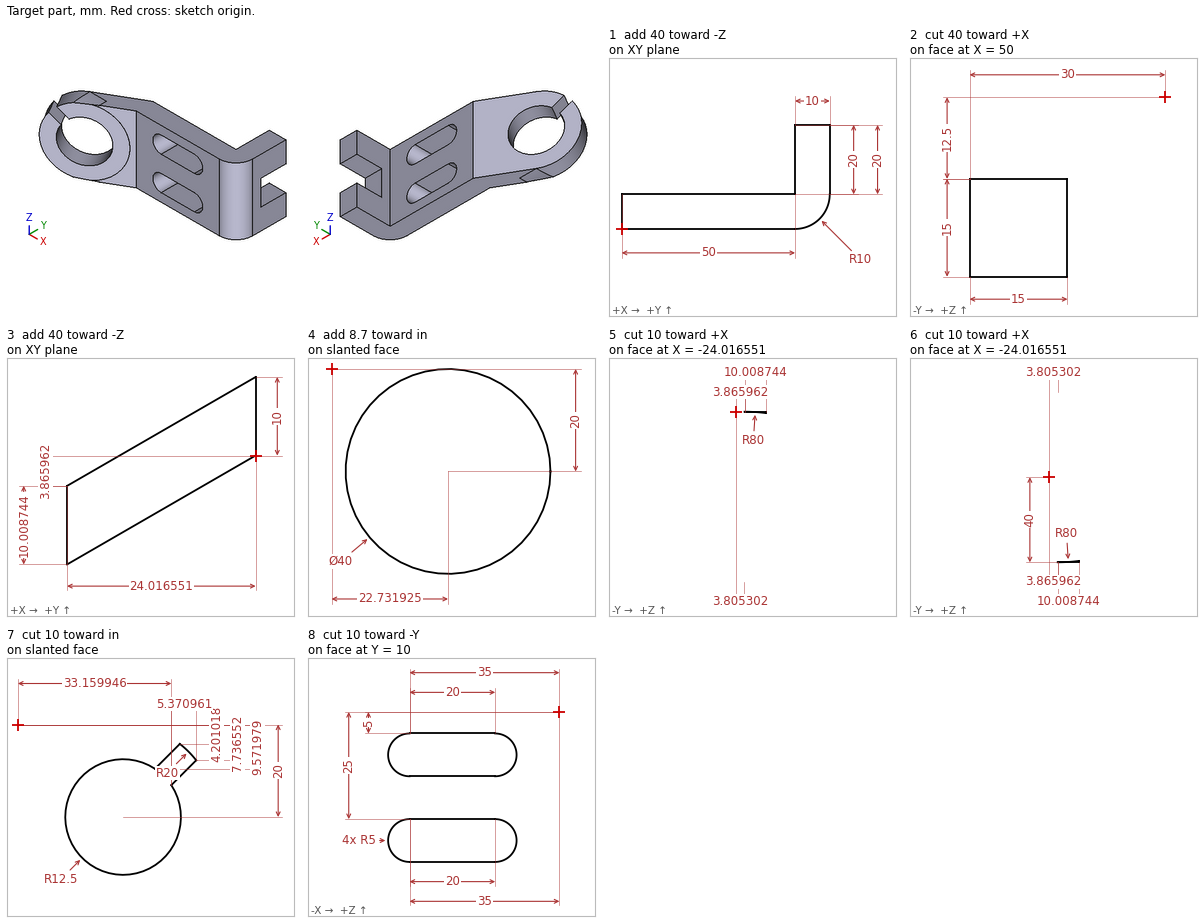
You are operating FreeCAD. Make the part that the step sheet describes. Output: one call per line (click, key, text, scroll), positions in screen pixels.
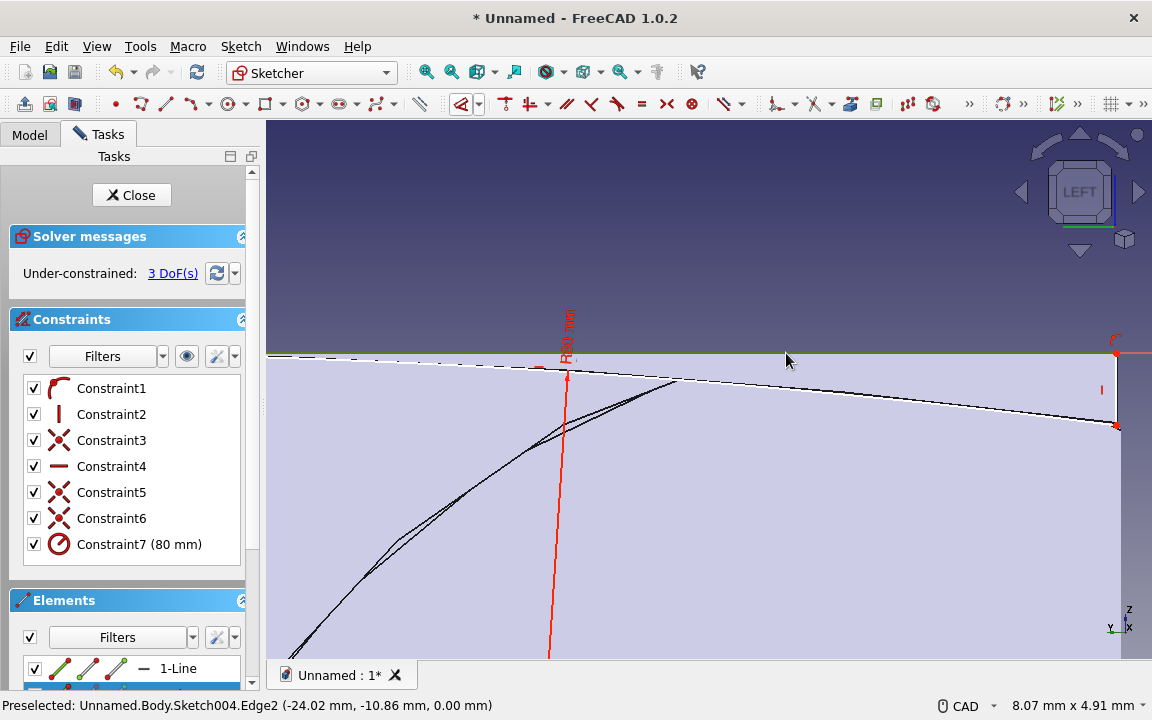
key(l)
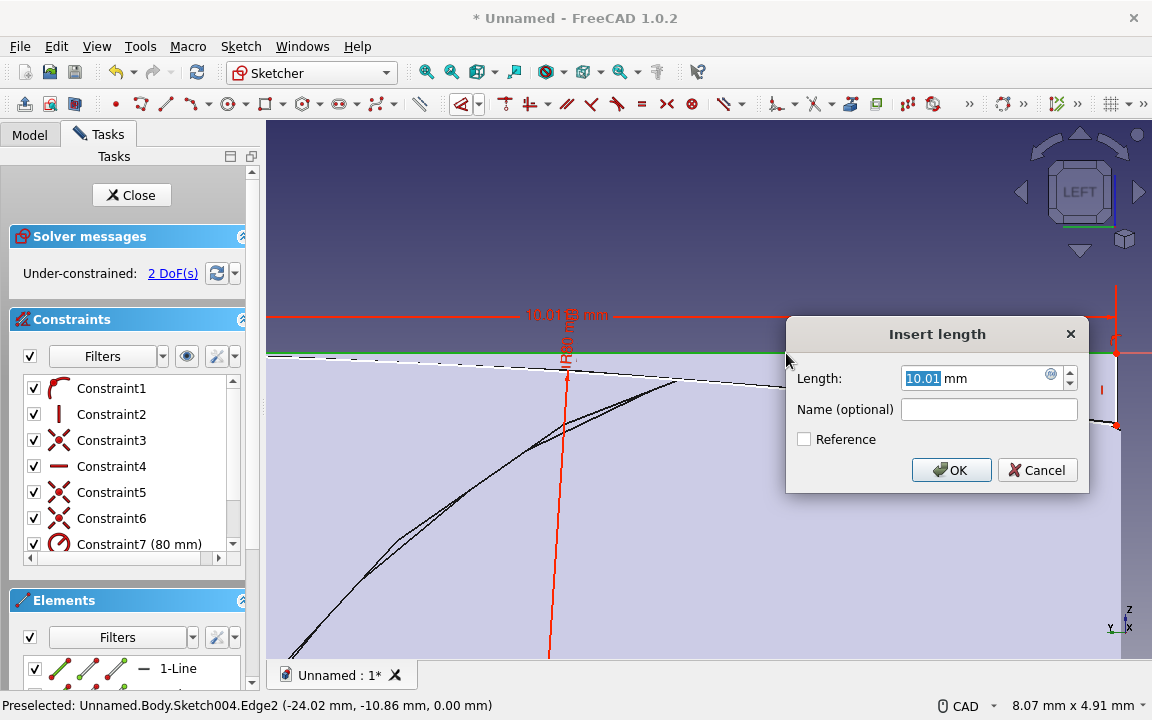
text(10.008744)
key(Return)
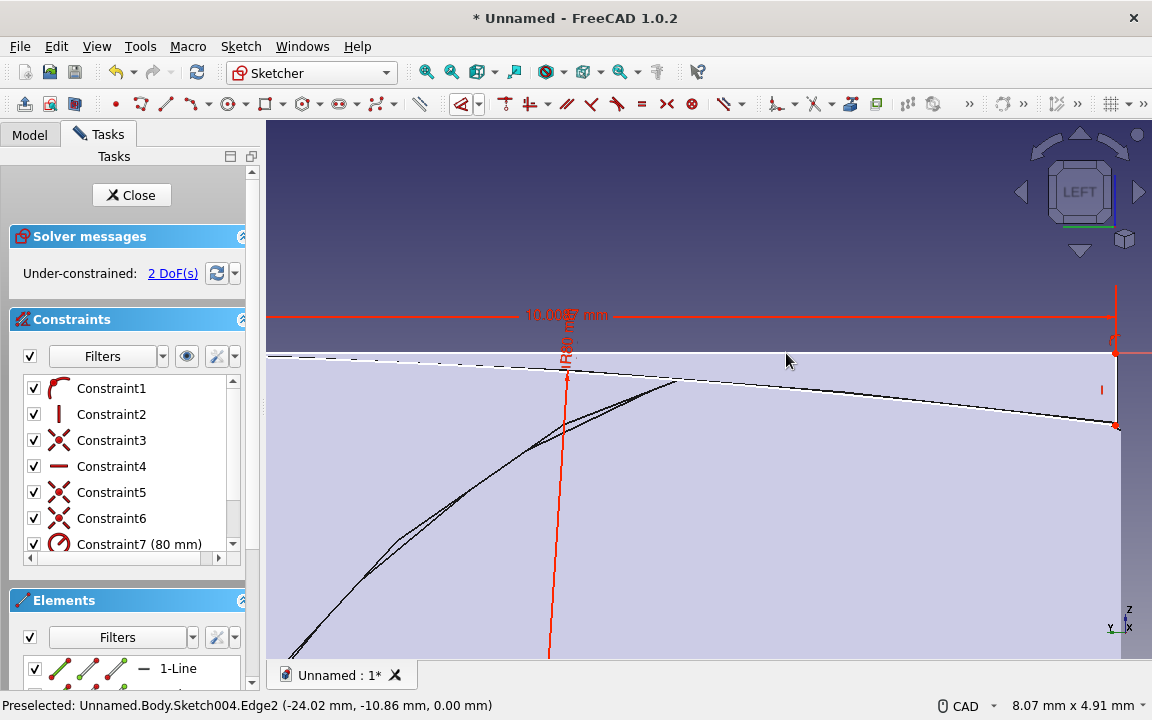
scroll(764, 390, down, 6)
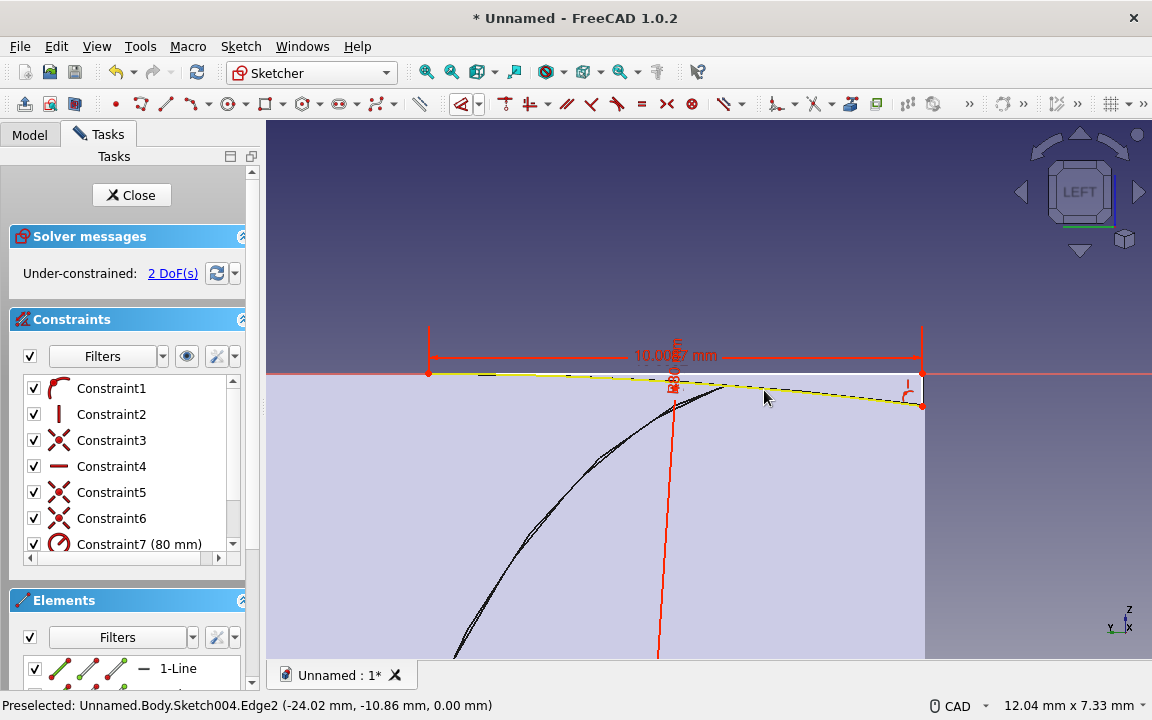
click(539, 379)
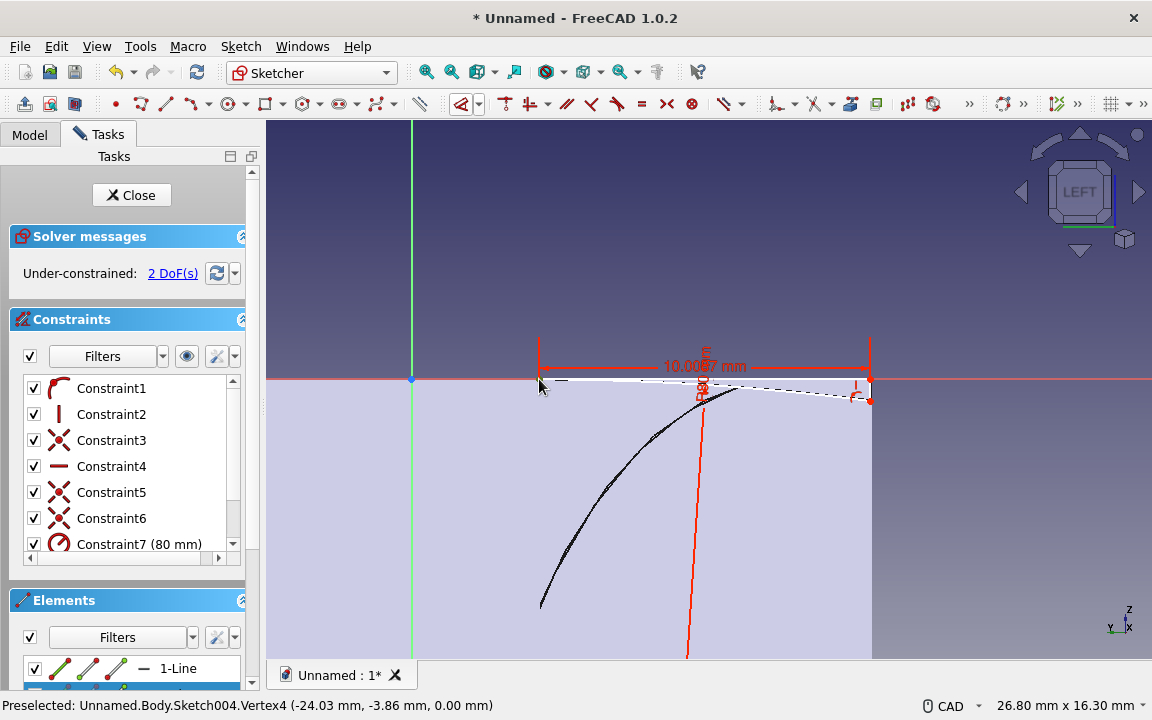
click(478, 104)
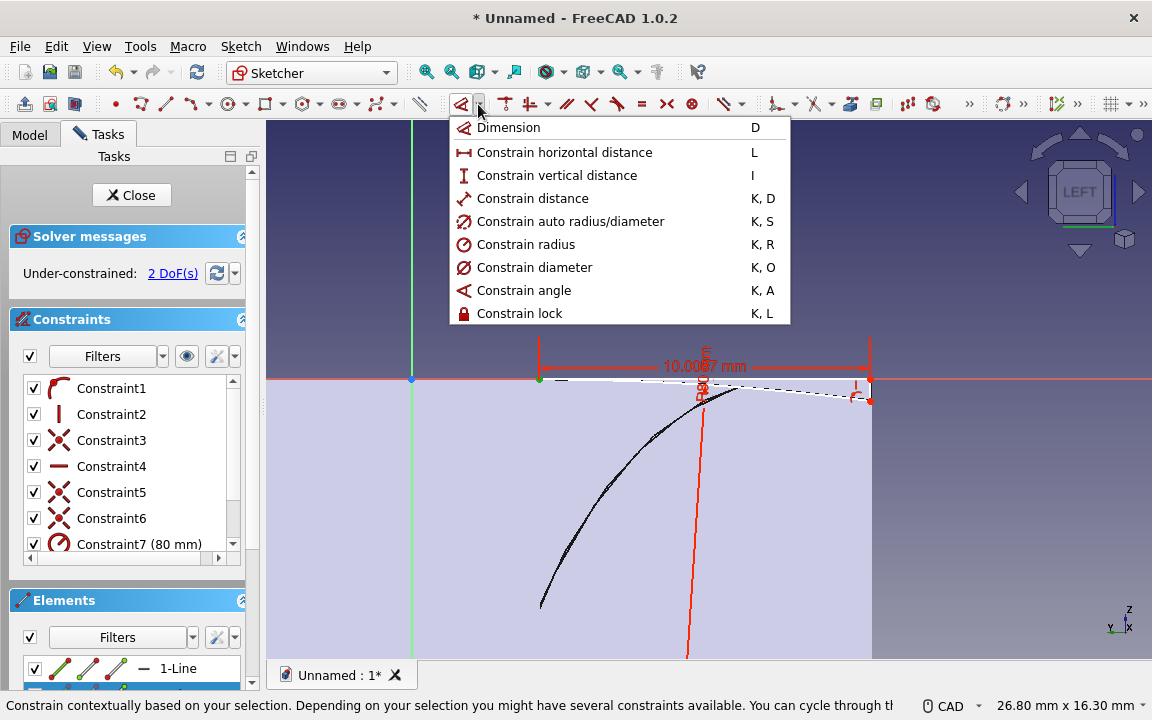
click(620, 152)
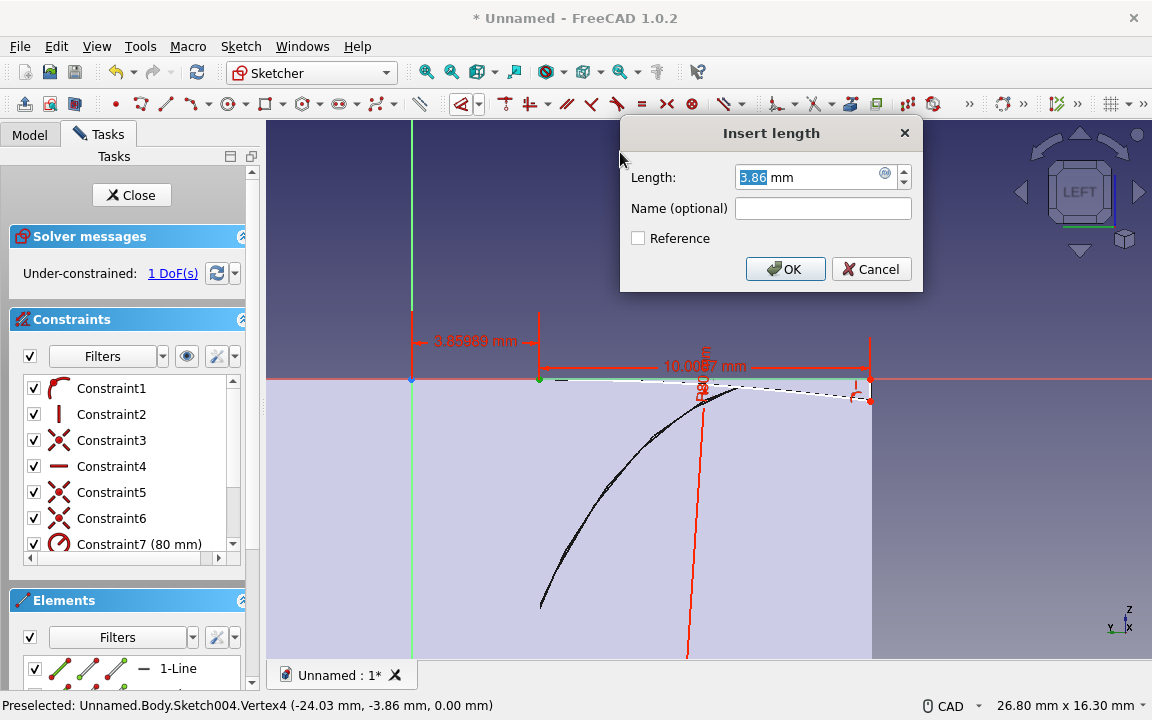
text(3.865962)
key(Return)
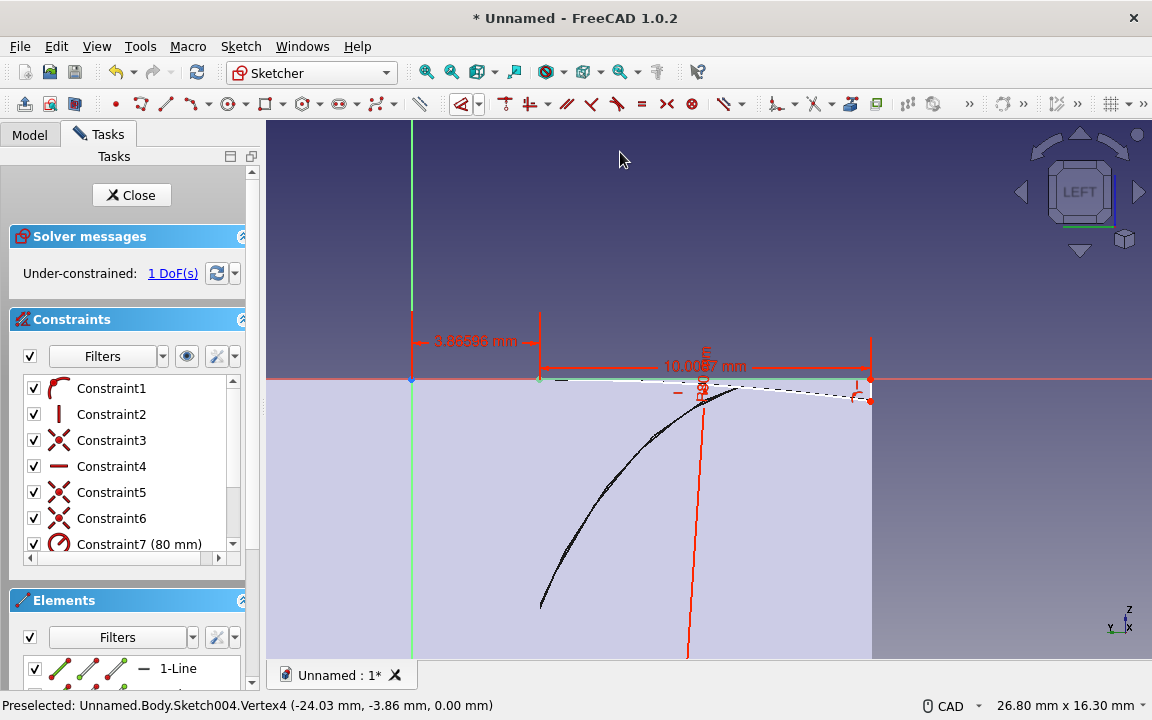
scroll(640, 184, down, 10)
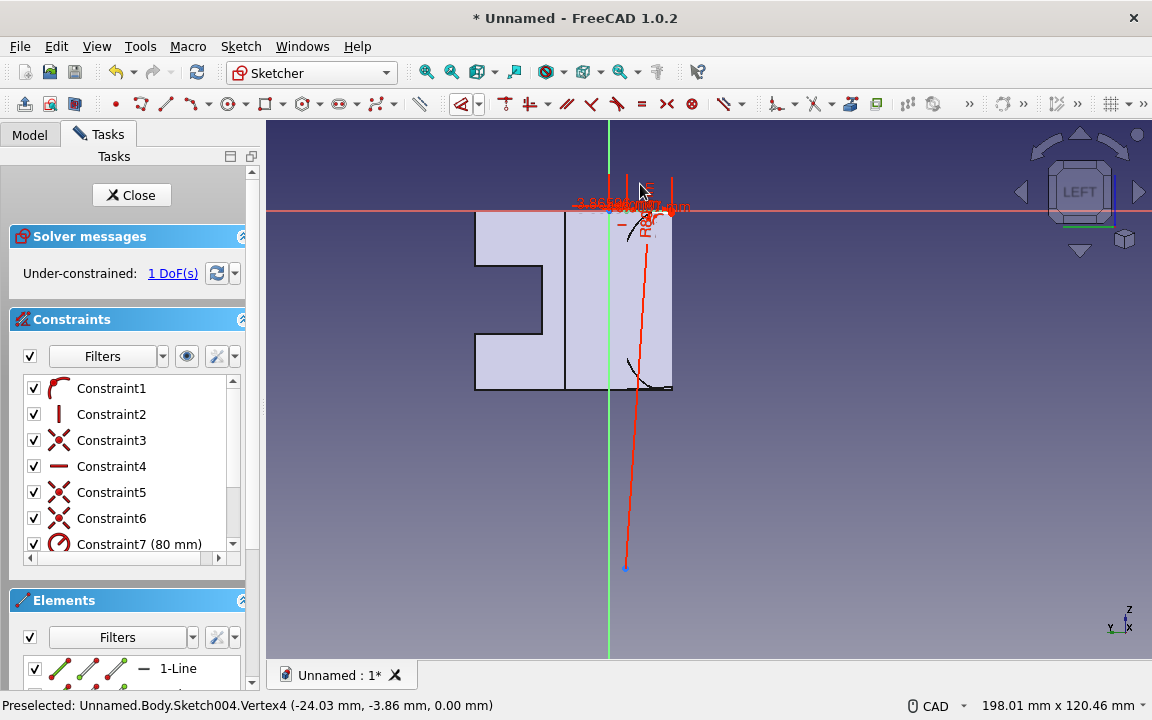
scroll(626, 568, up, 5)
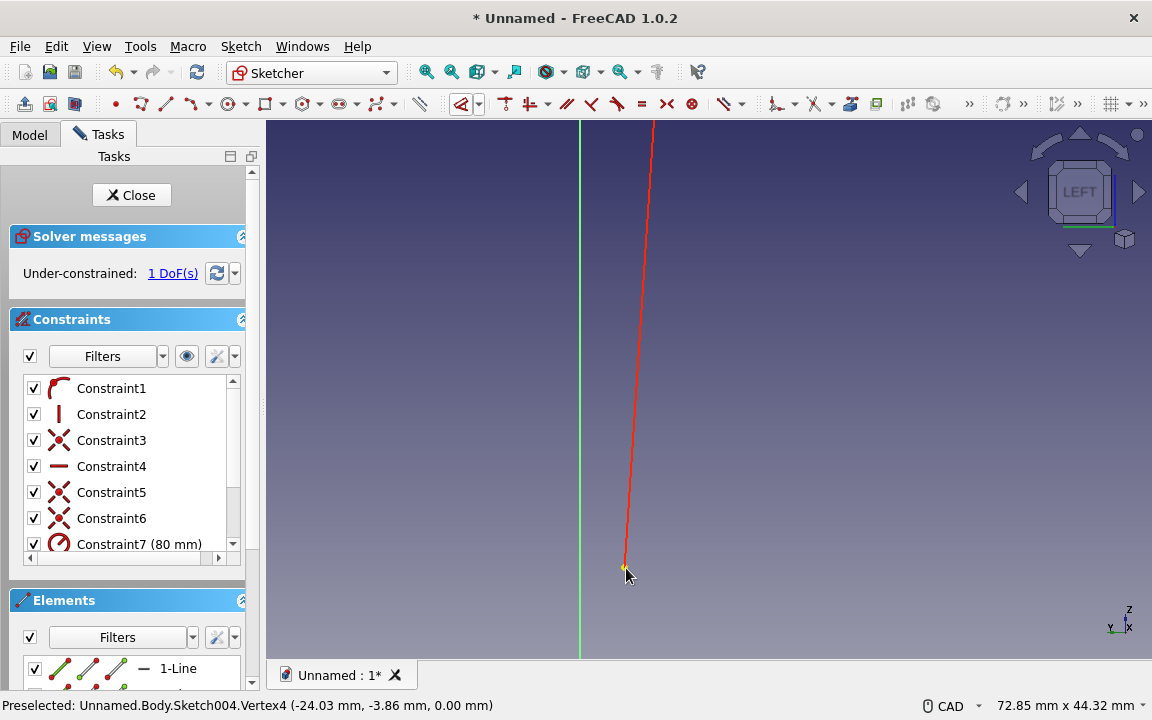
click(625, 568)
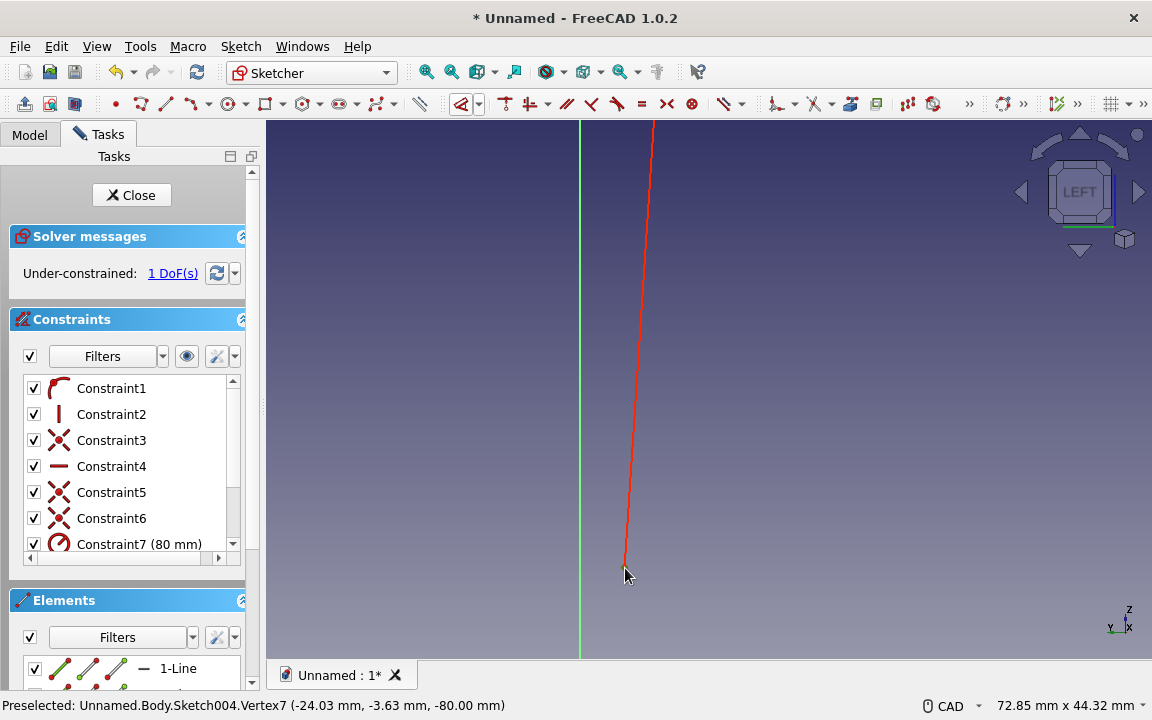
key(l)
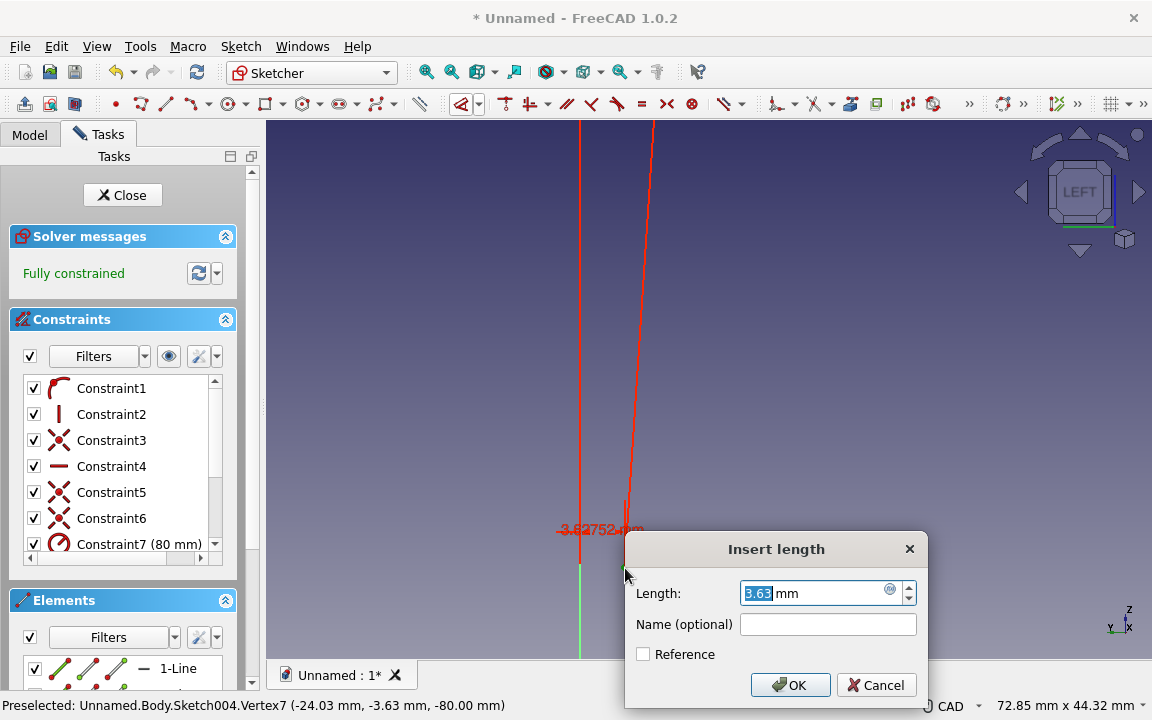
text(3.805302)
key(Return)